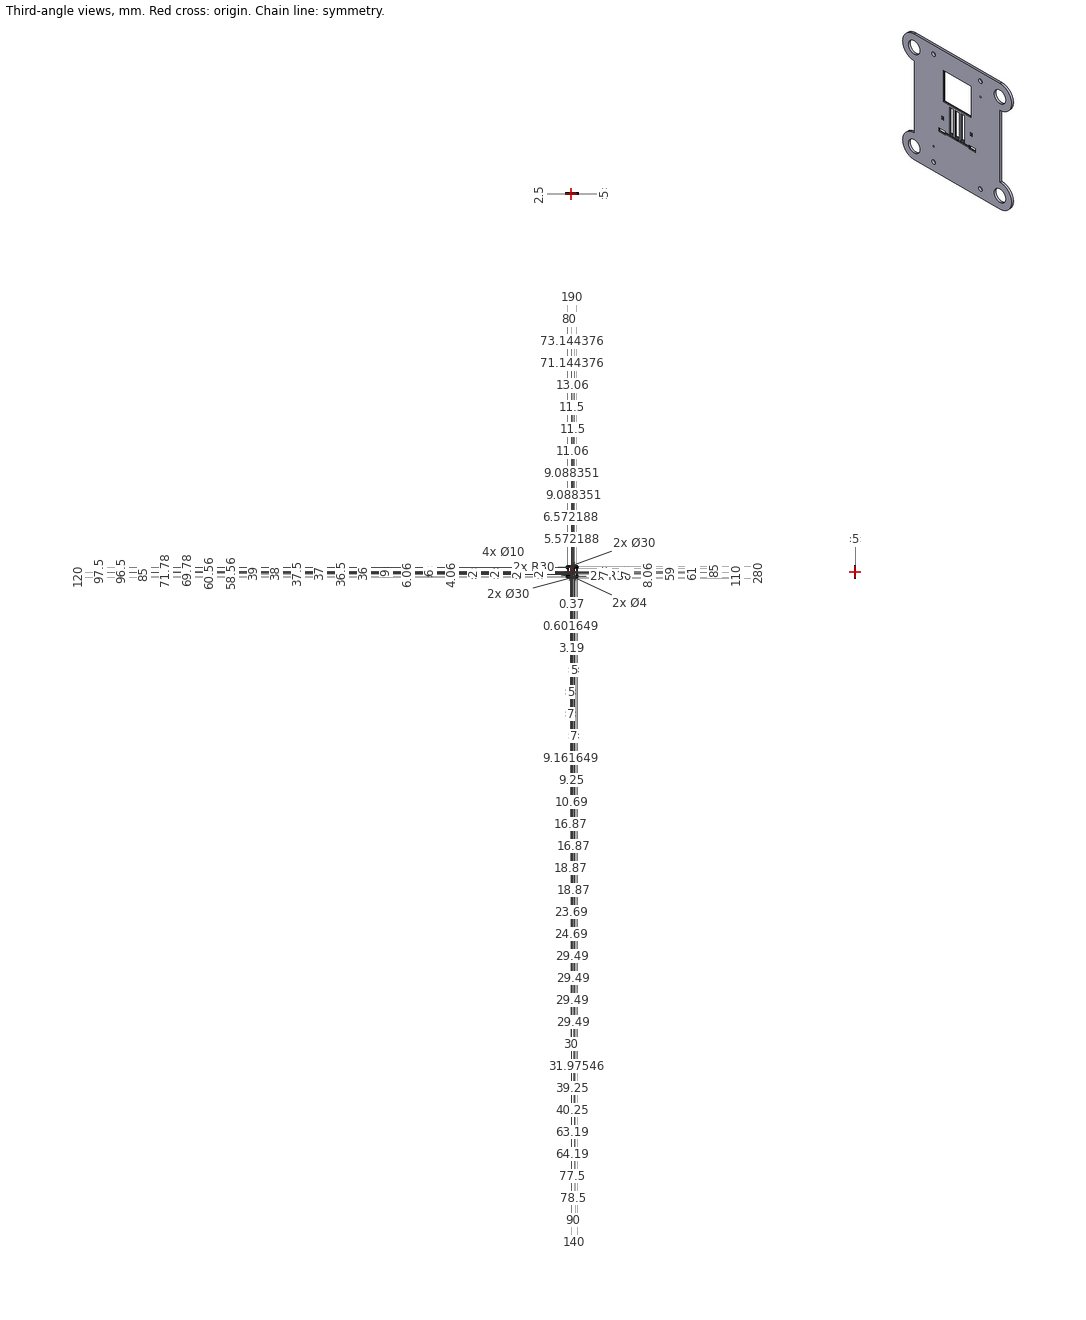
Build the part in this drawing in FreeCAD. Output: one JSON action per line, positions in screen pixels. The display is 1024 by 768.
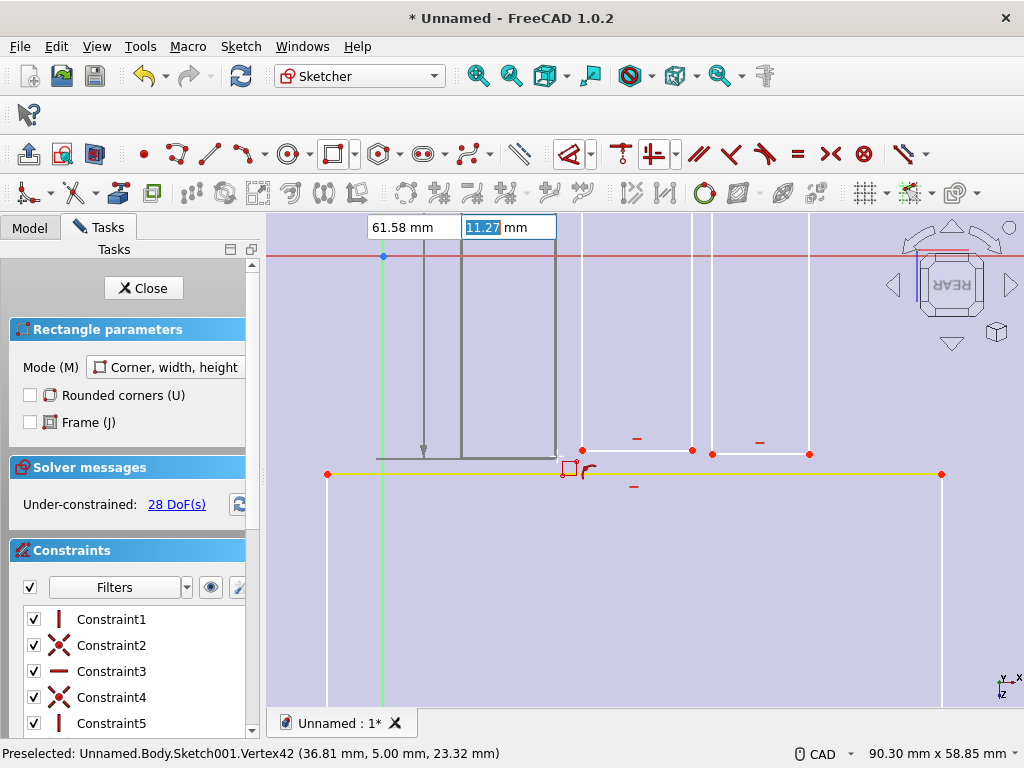
{"action": "left_click", "coordinate": [558, 453]}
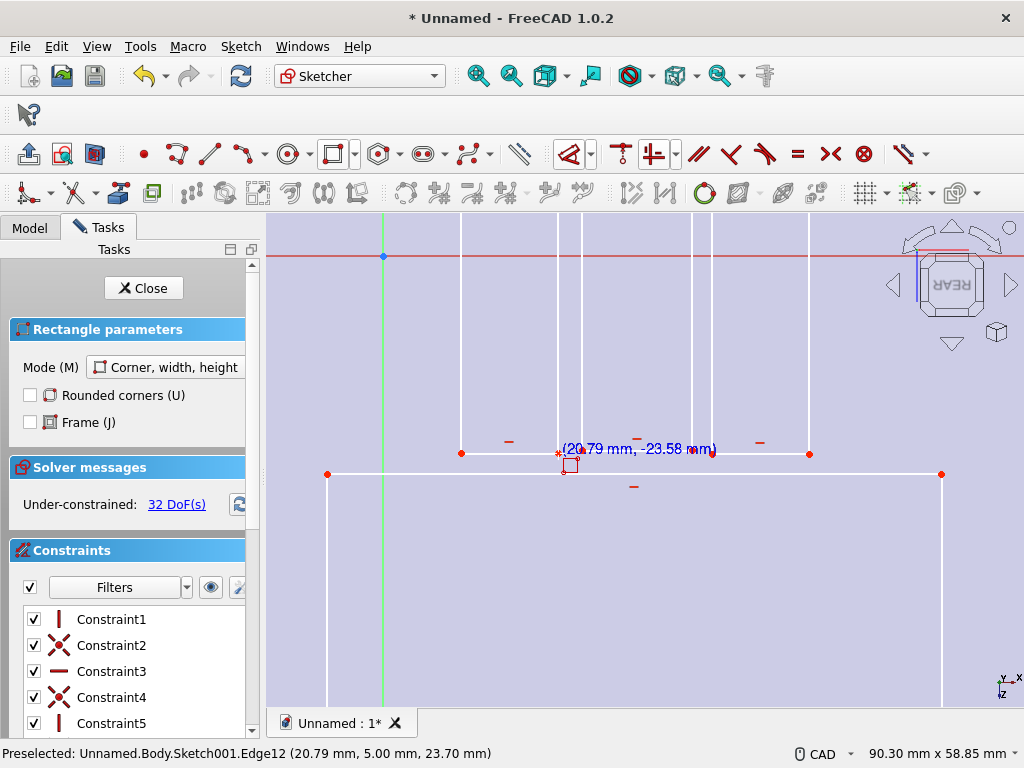
{"action": "left_click", "coordinate": [177, 154]}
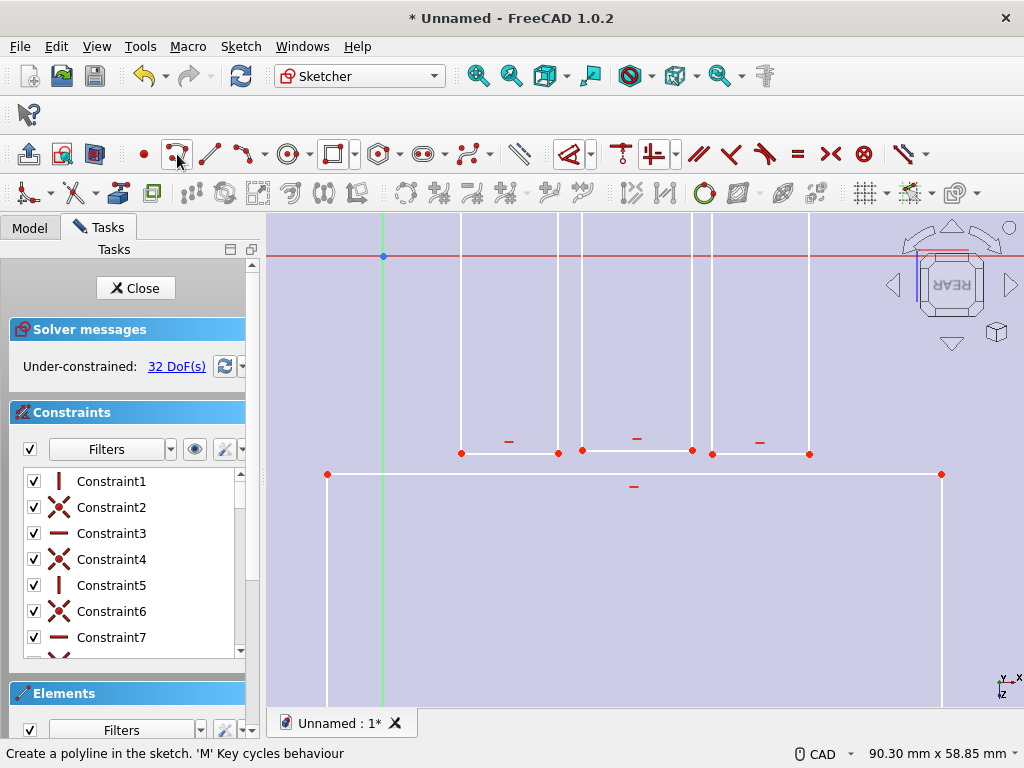
{"action": "scroll", "coordinate": [557, 456], "scroll_direction": "down", "scroll_amount": 7}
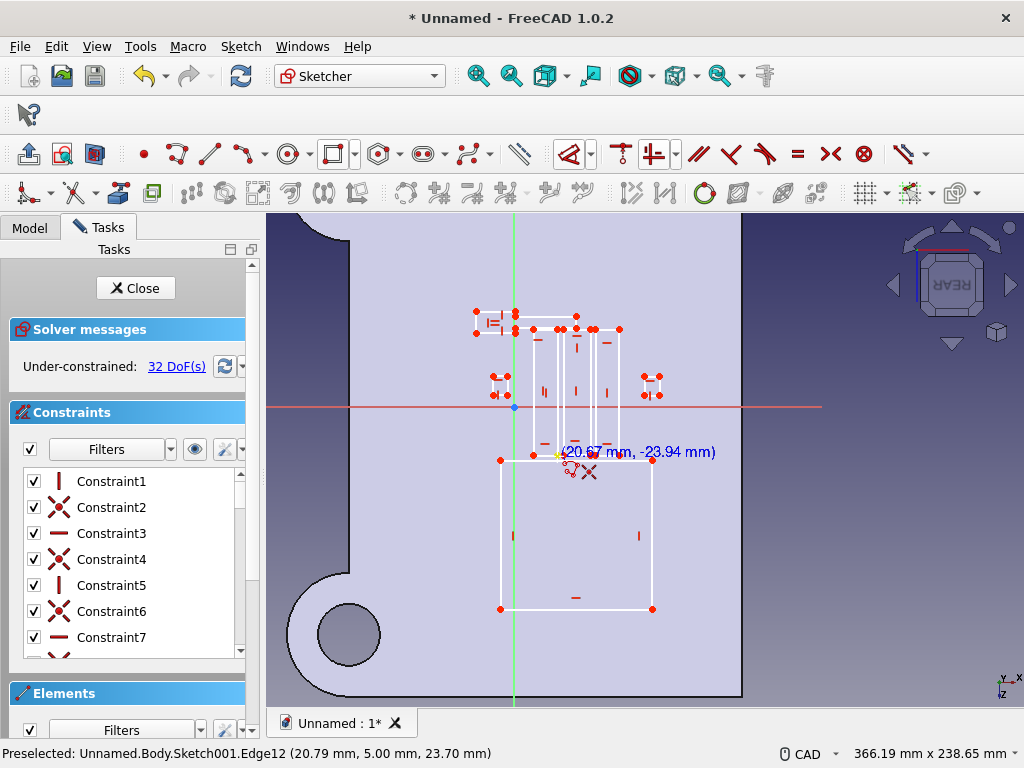
{"action": "scroll", "coordinate": [577, 328], "scroll_direction": "up", "scroll_amount": 17}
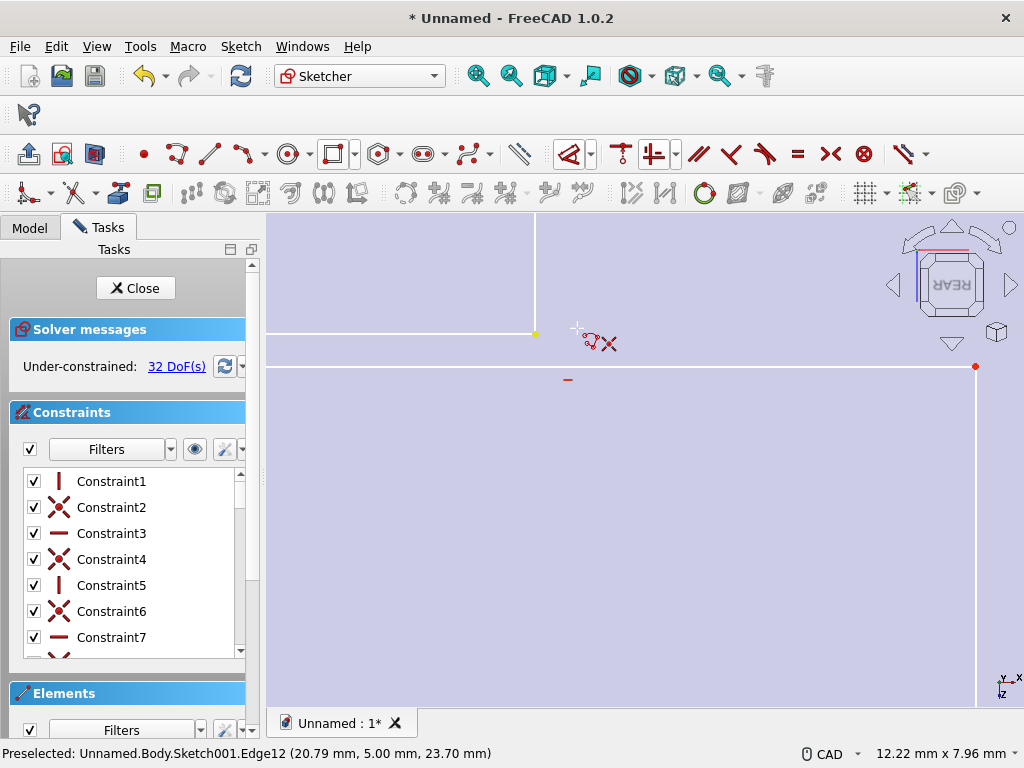
{"action": "left_click", "coordinate": [562, 334]}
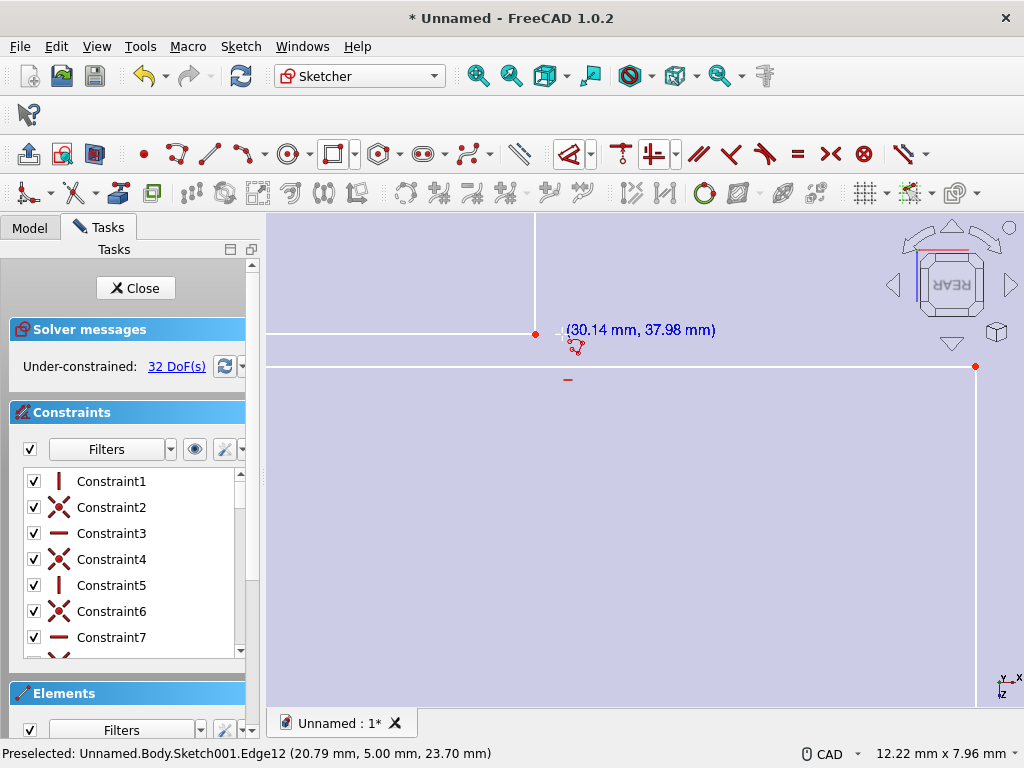
{"action": "scroll", "coordinate": [577, 297], "scroll_direction": "down", "scroll_amount": 16}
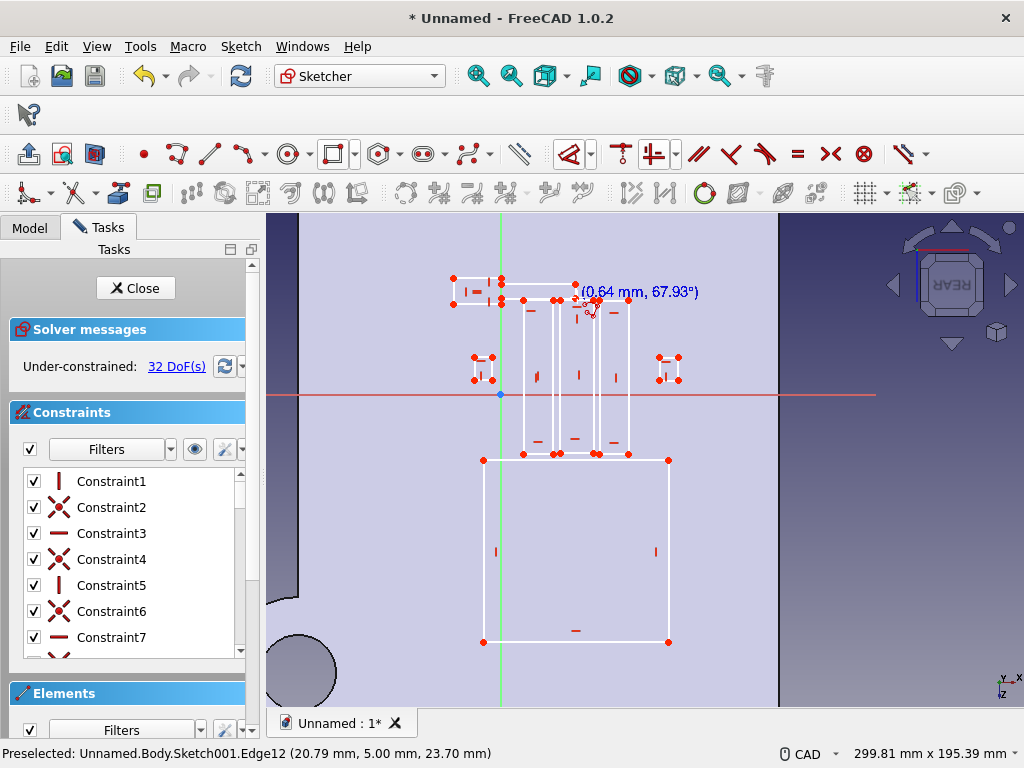
{"action": "left_click", "coordinate": [651, 299]}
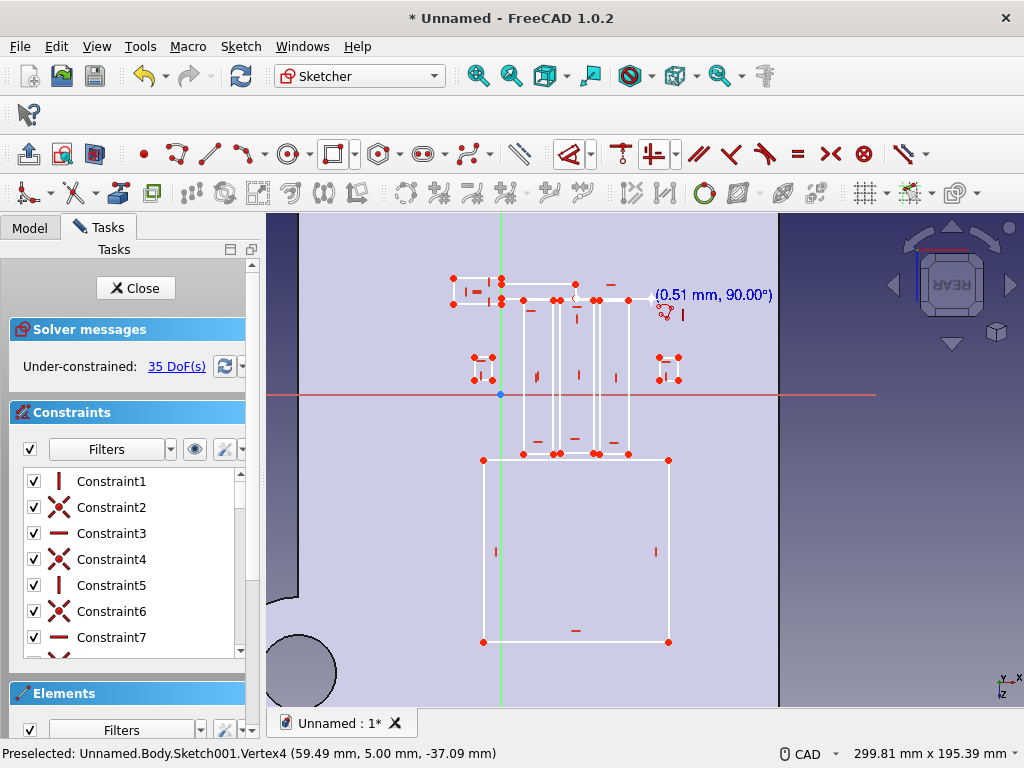
{"action": "scroll", "coordinate": [651, 304], "scroll_direction": "up", "scroll_amount": 6}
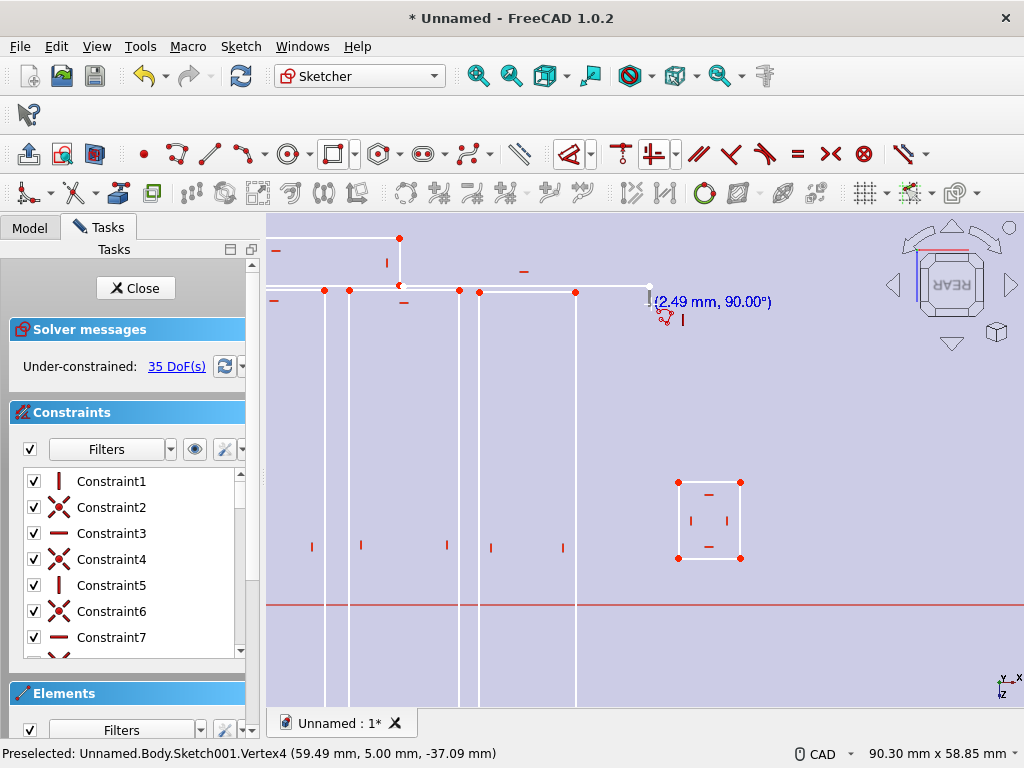
{"action": "left_click", "coordinate": [650, 303]}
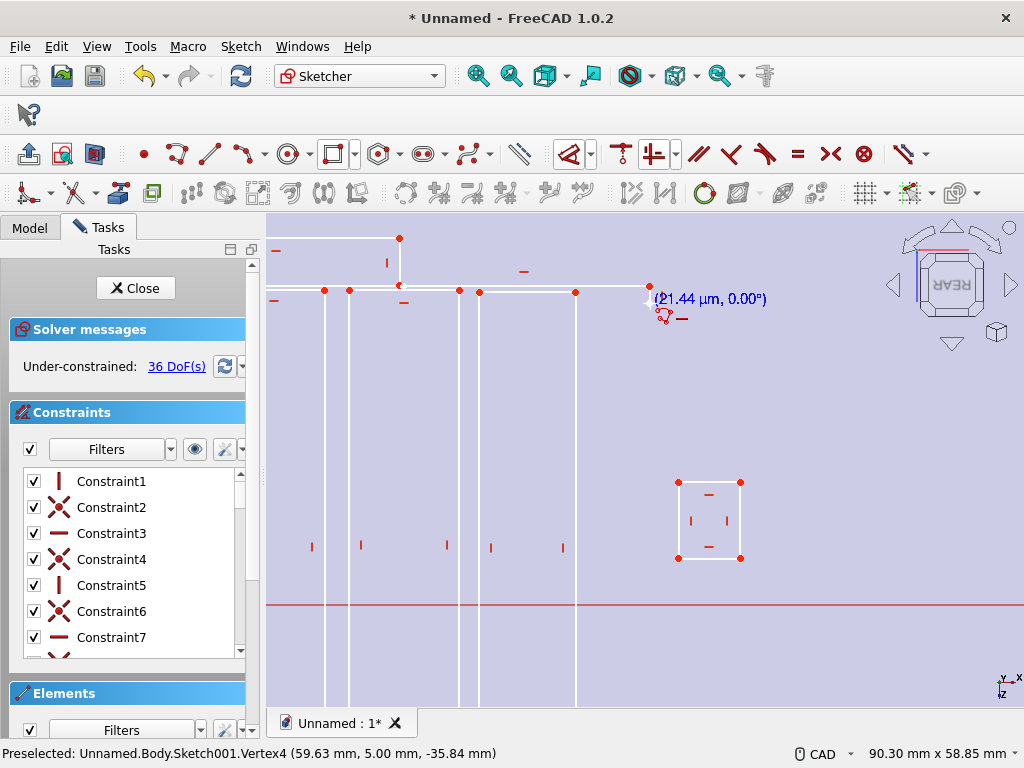
{"action": "scroll", "coordinate": [634, 342], "scroll_direction": "down", "scroll_amount": 7}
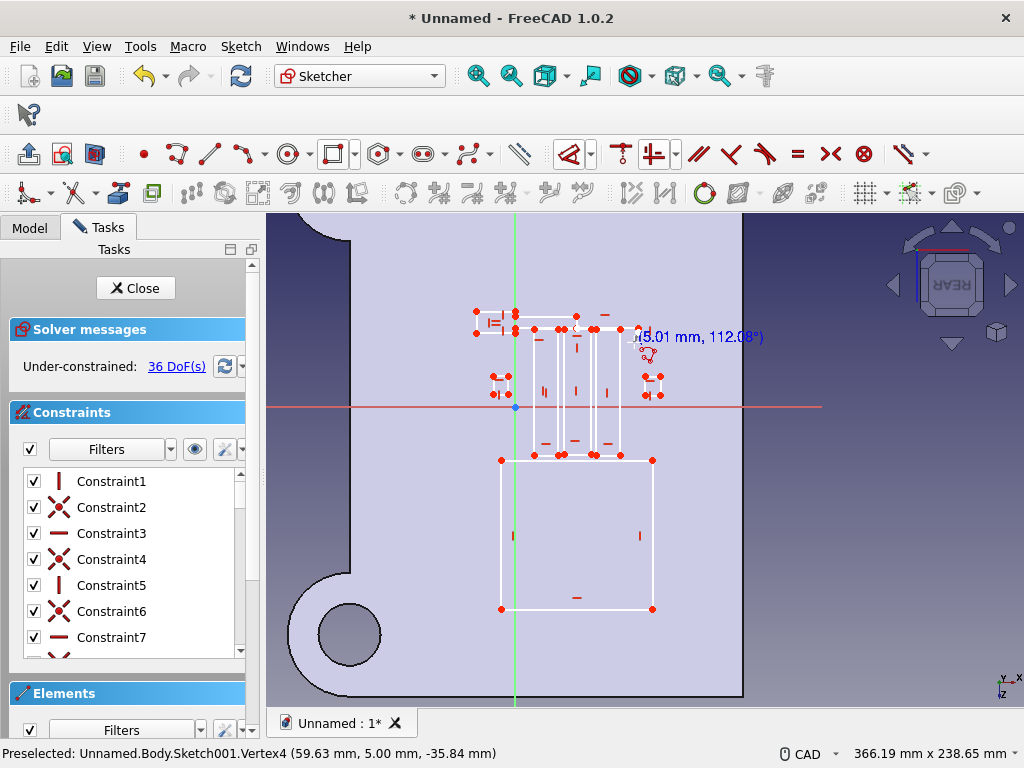
{"action": "left_click", "coordinate": [678, 333]}
{"action": "left_click", "coordinate": [678, 312]}
{"action": "left_click", "coordinate": [639, 312]}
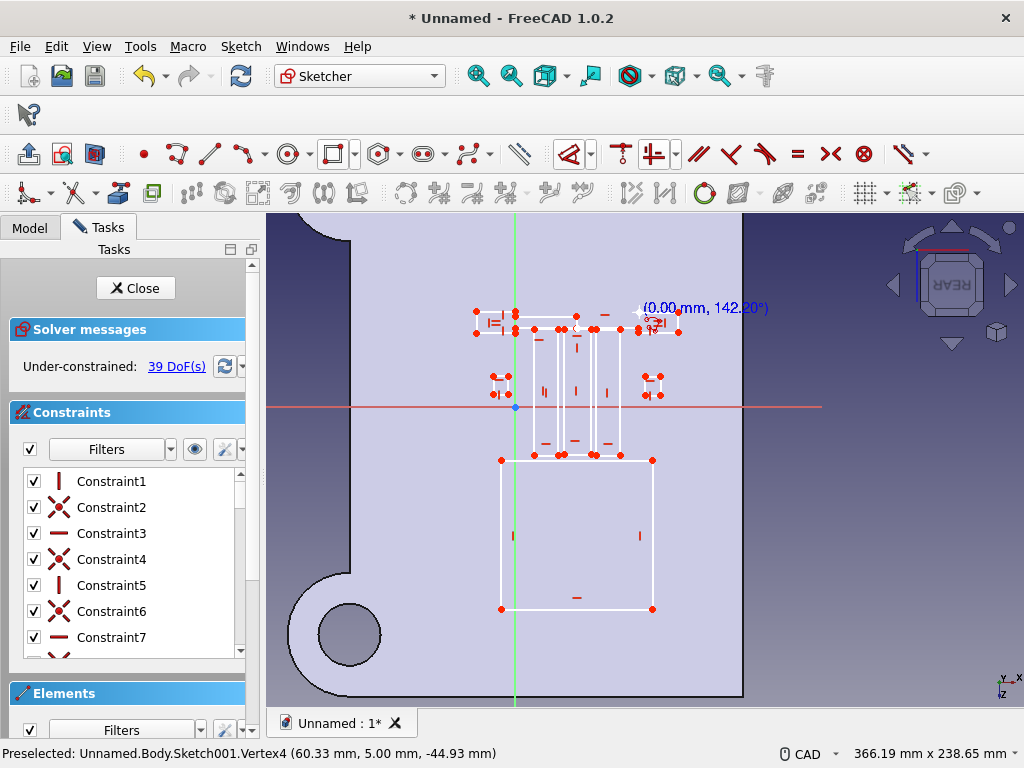
{"action": "scroll", "coordinate": [639, 316], "scroll_direction": "up", "scroll_amount": 7}